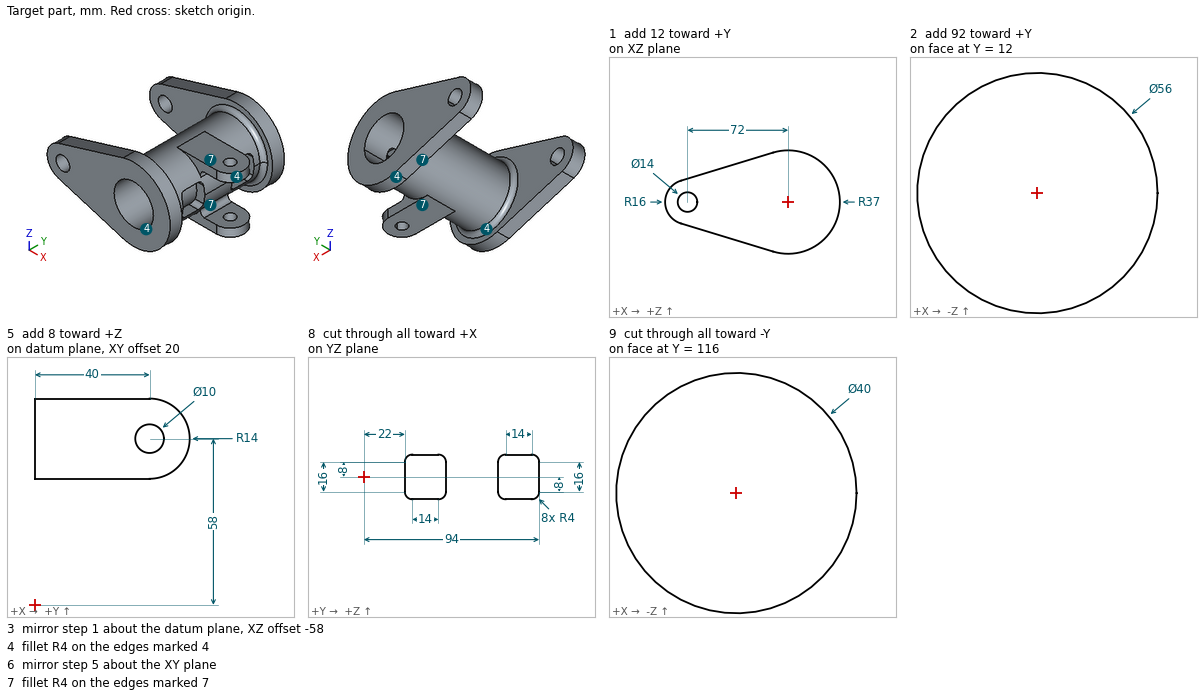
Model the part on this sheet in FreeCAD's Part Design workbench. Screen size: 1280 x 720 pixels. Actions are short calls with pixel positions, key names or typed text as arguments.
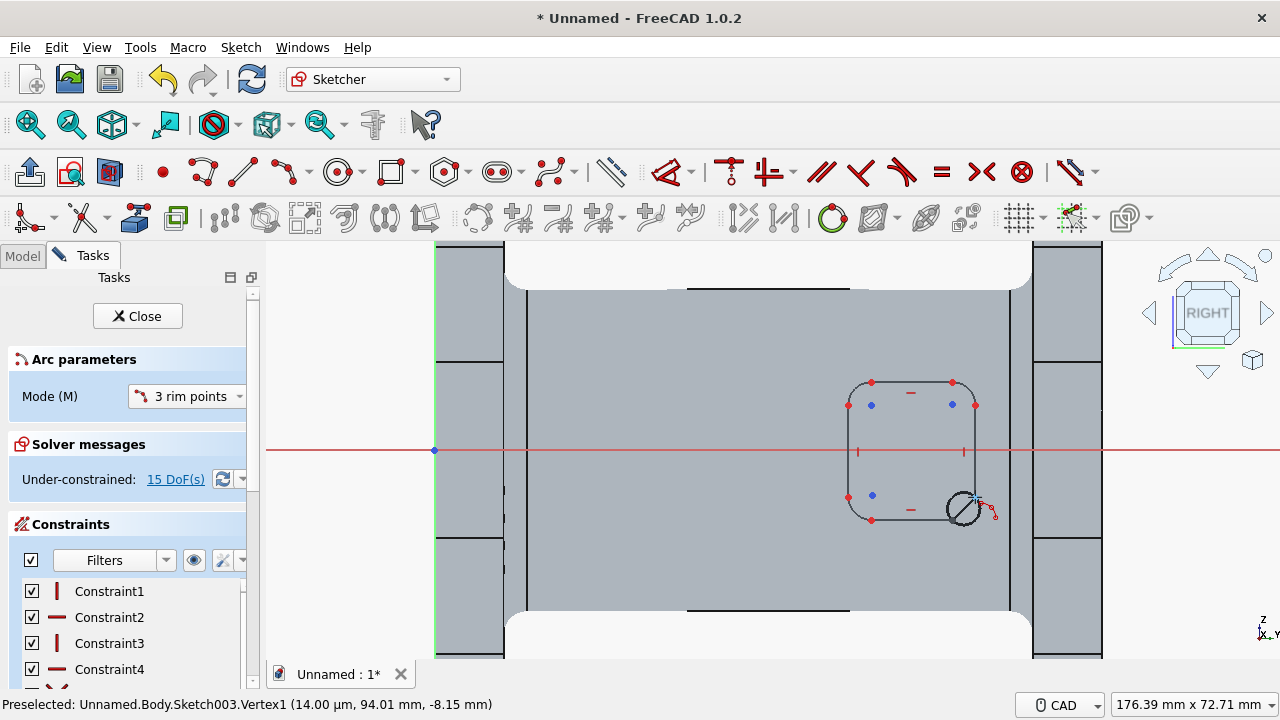
scroll(968, 513, up, 5)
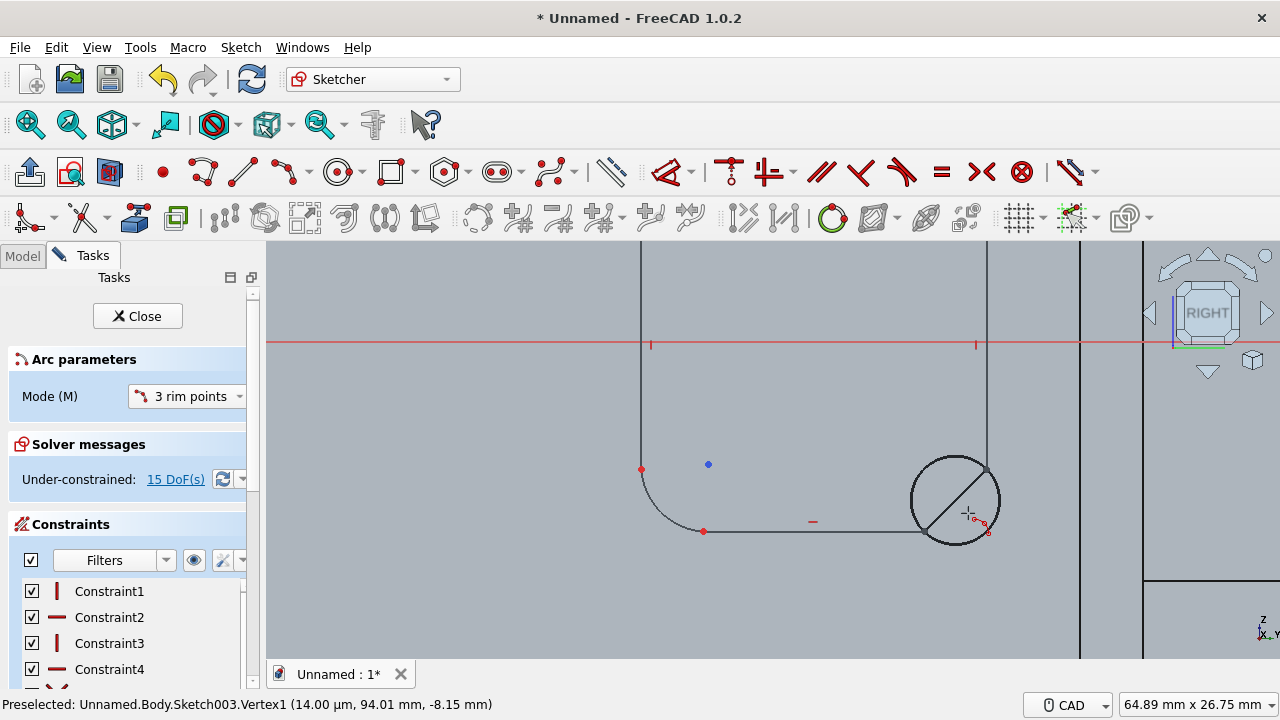
click(968, 511)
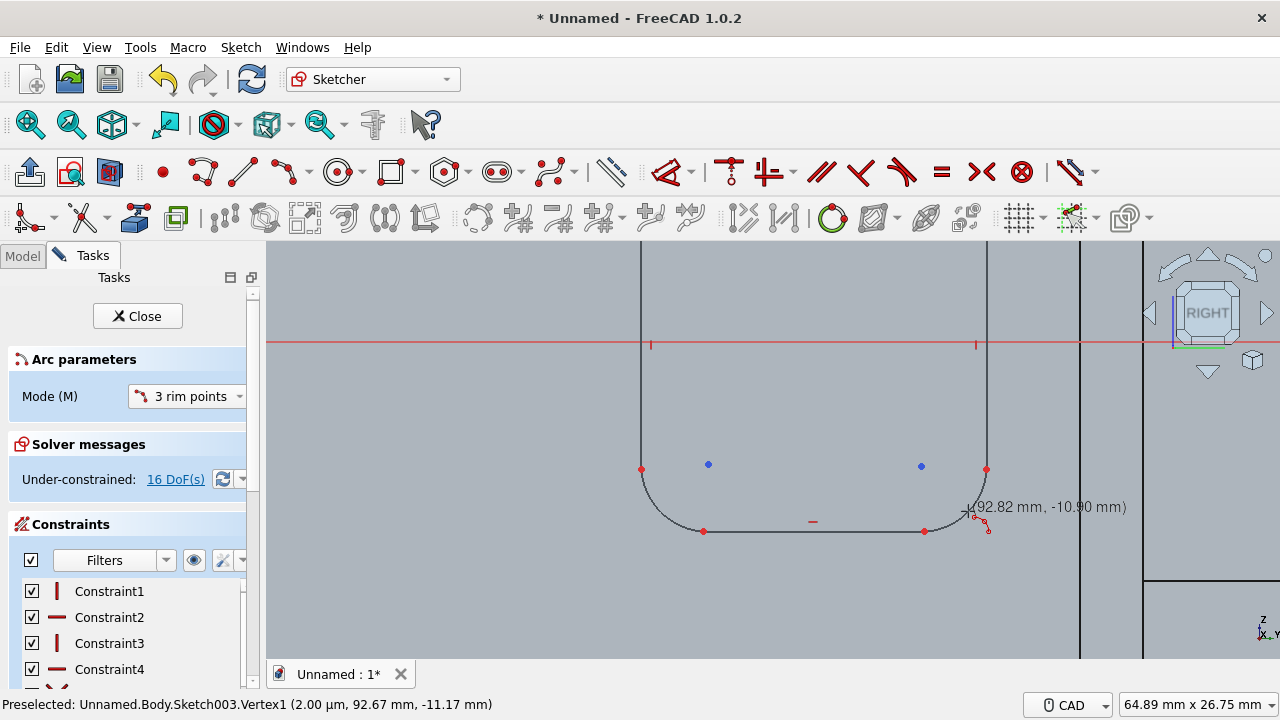
click(244, 172)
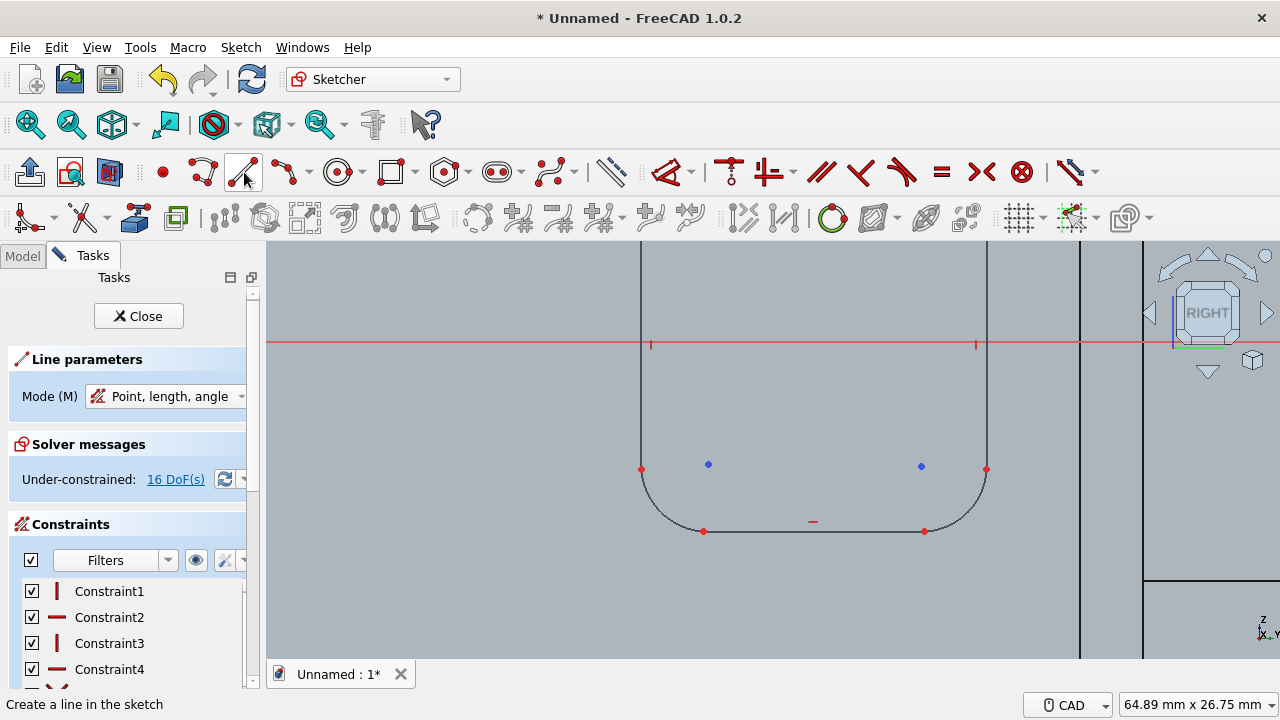
scroll(968, 513, down, 5)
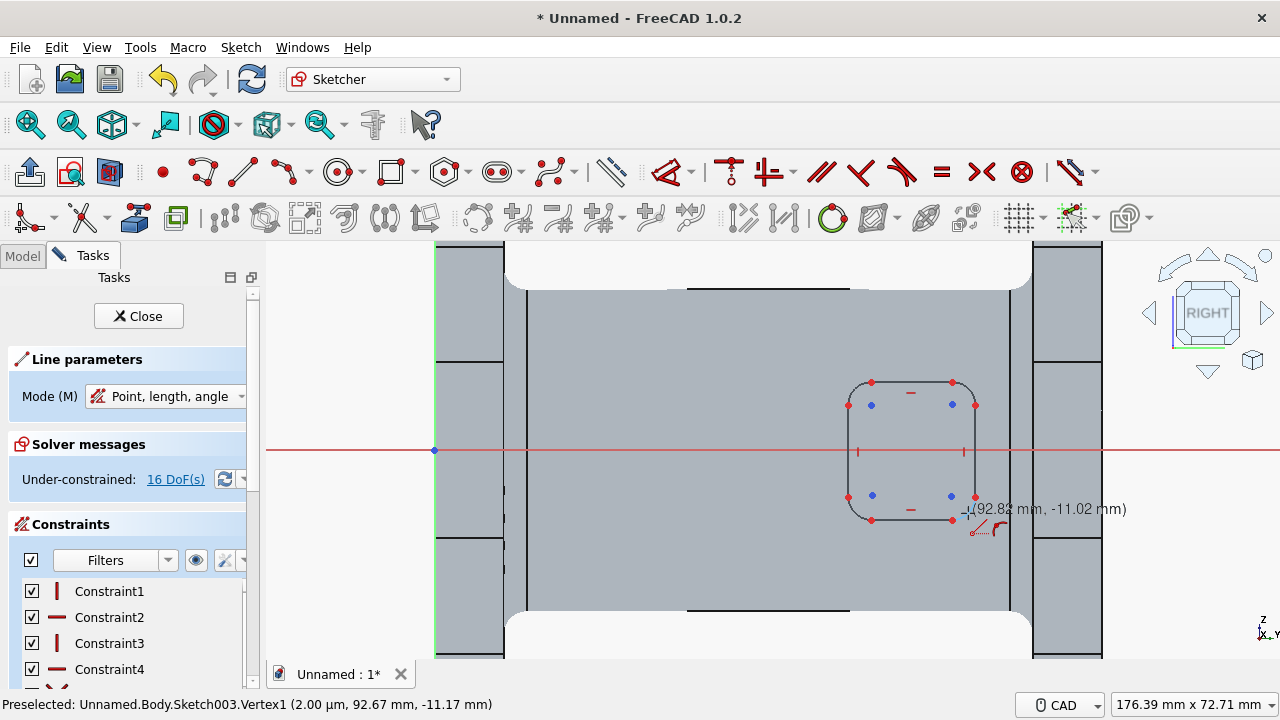
click(561, 404)
click(561, 496)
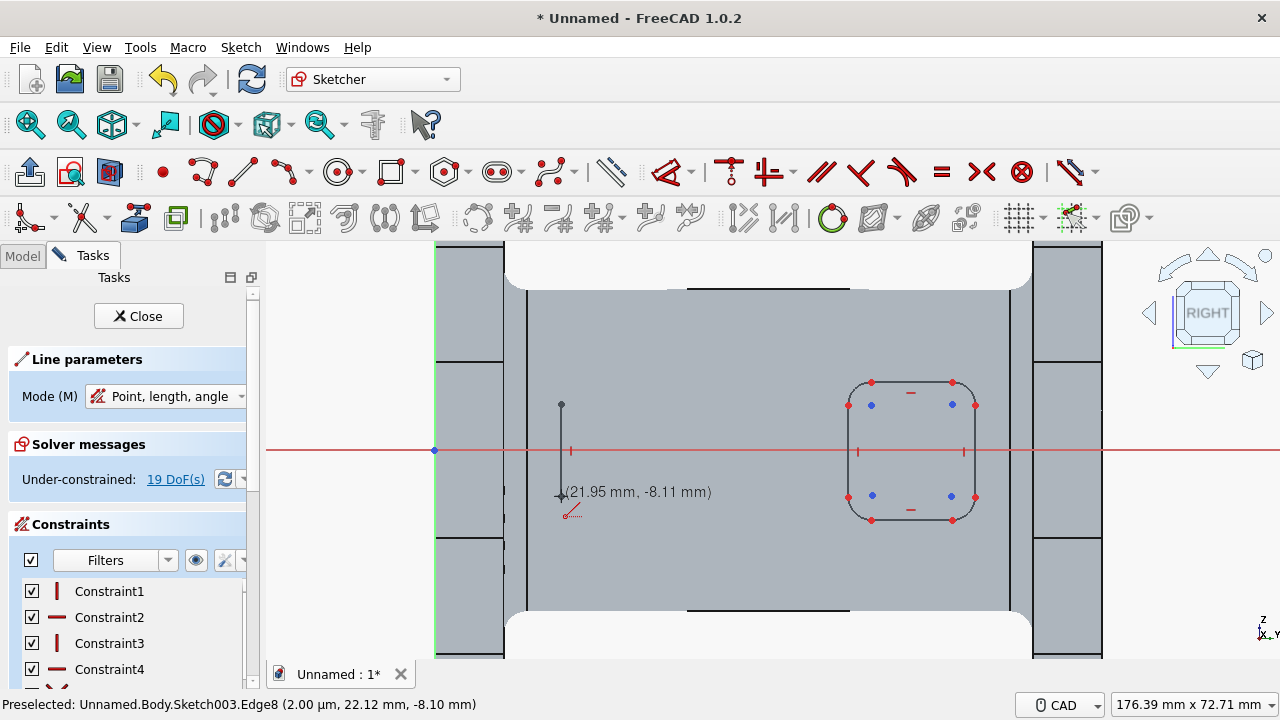
click(584, 519)
click(665, 519)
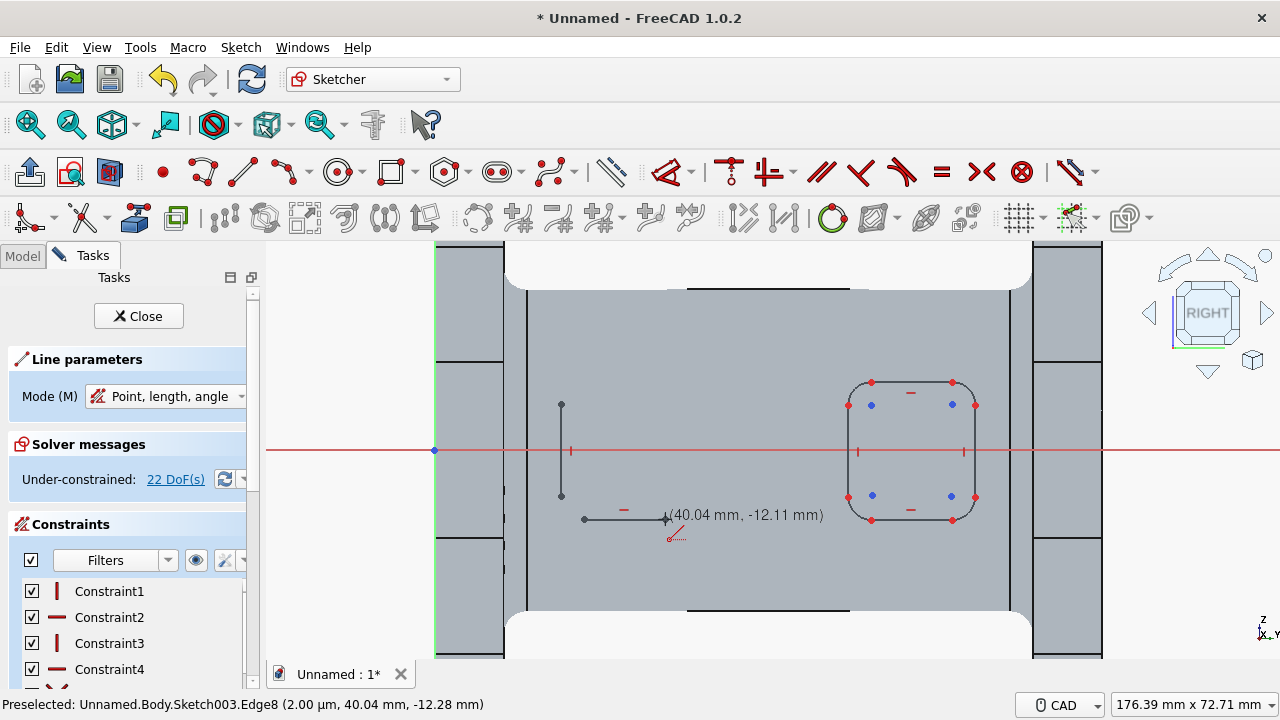
click(688, 496)
click(688, 404)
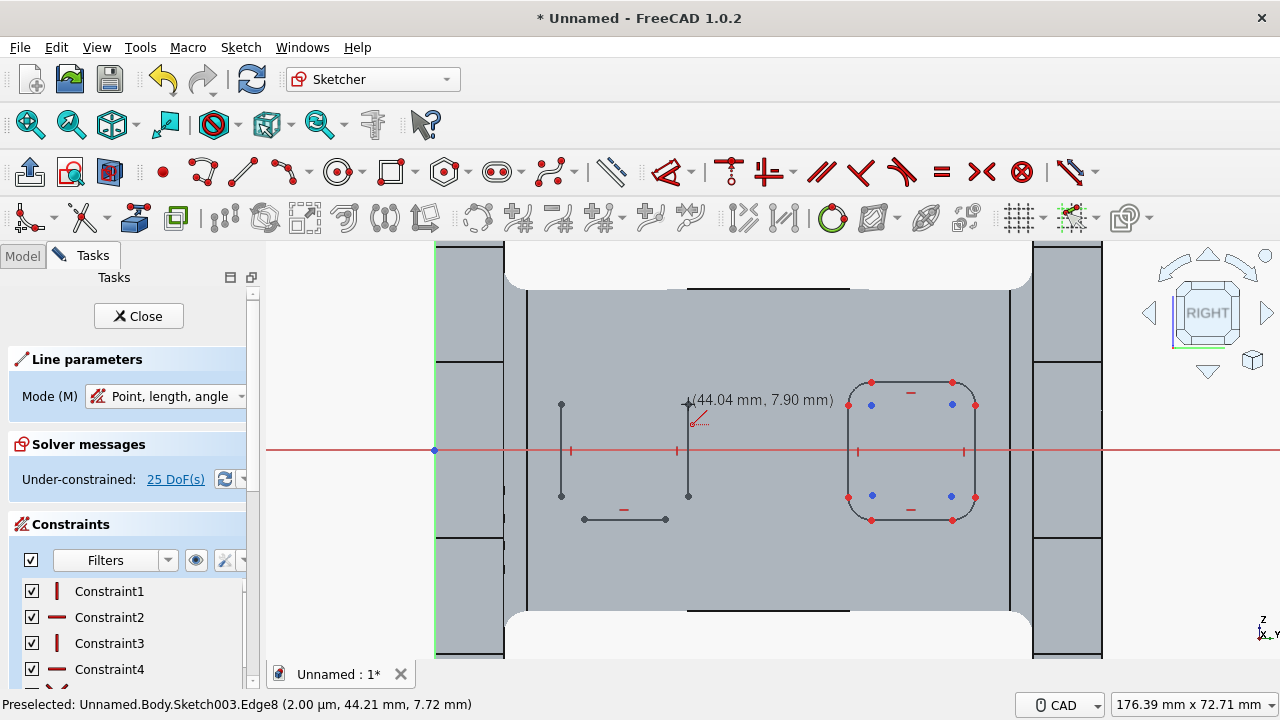
click(665, 381)
click(584, 381)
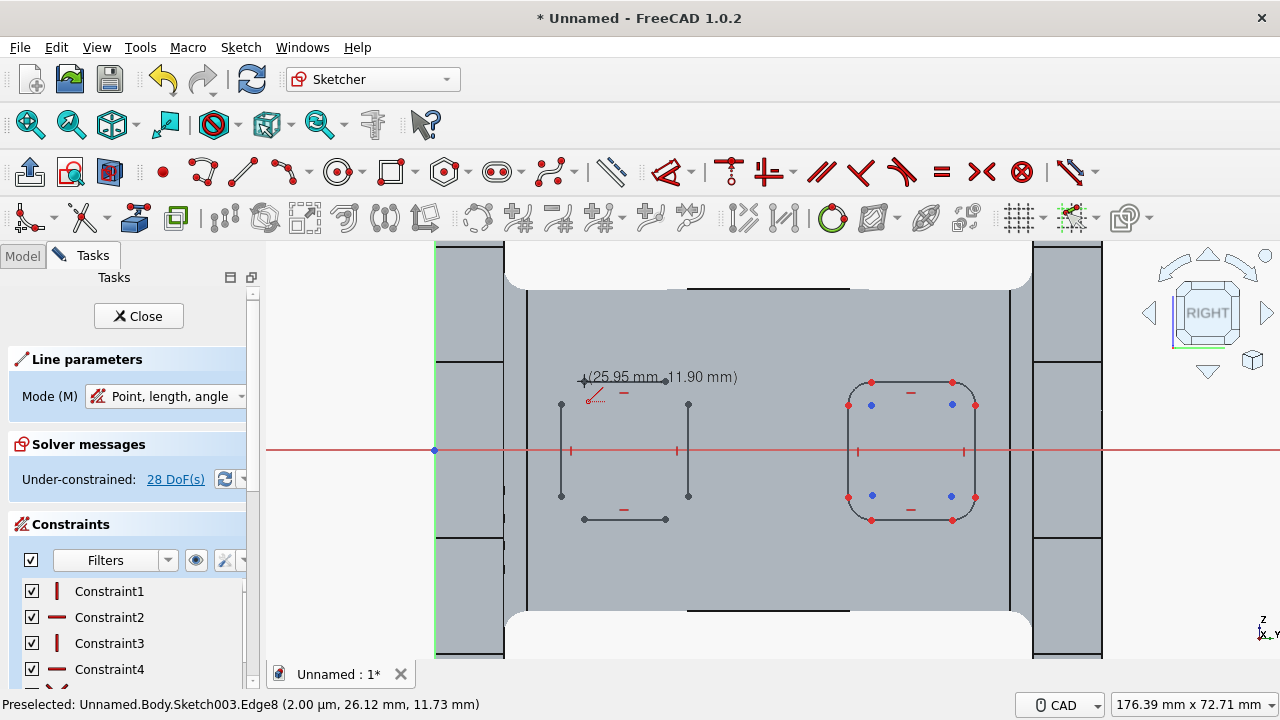
click(284, 172)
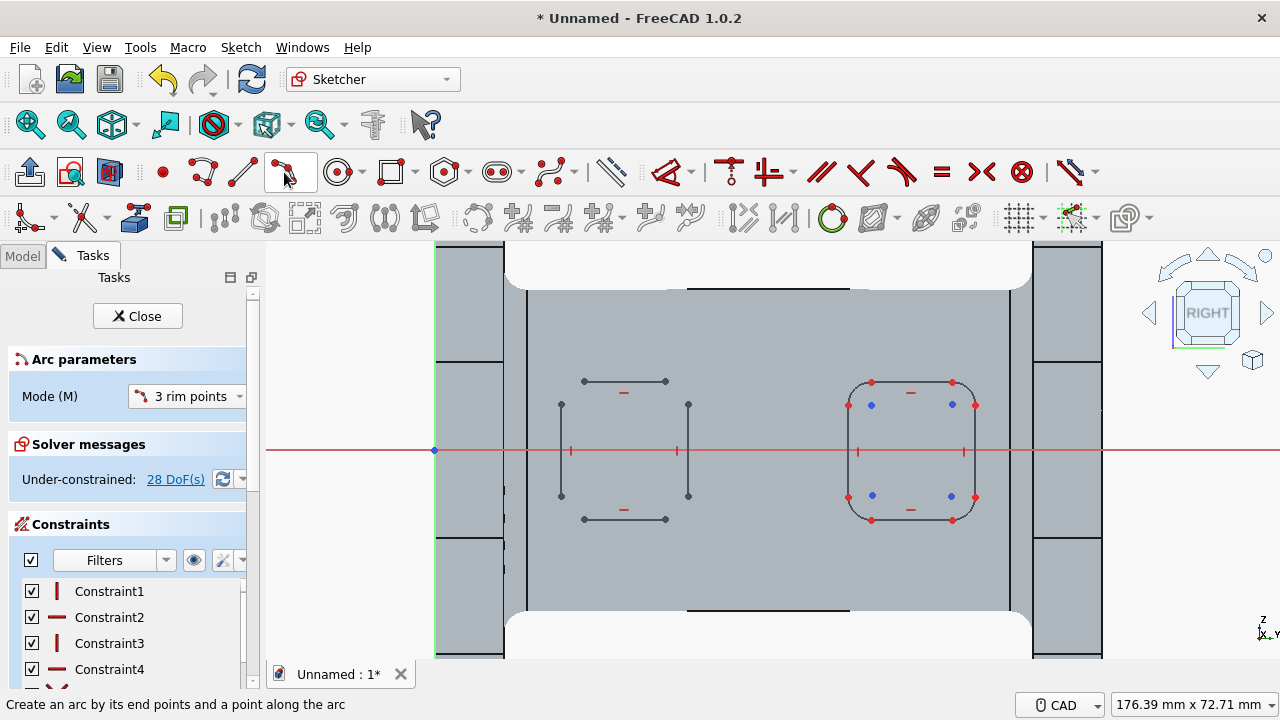
click(561, 497)
click(584, 520)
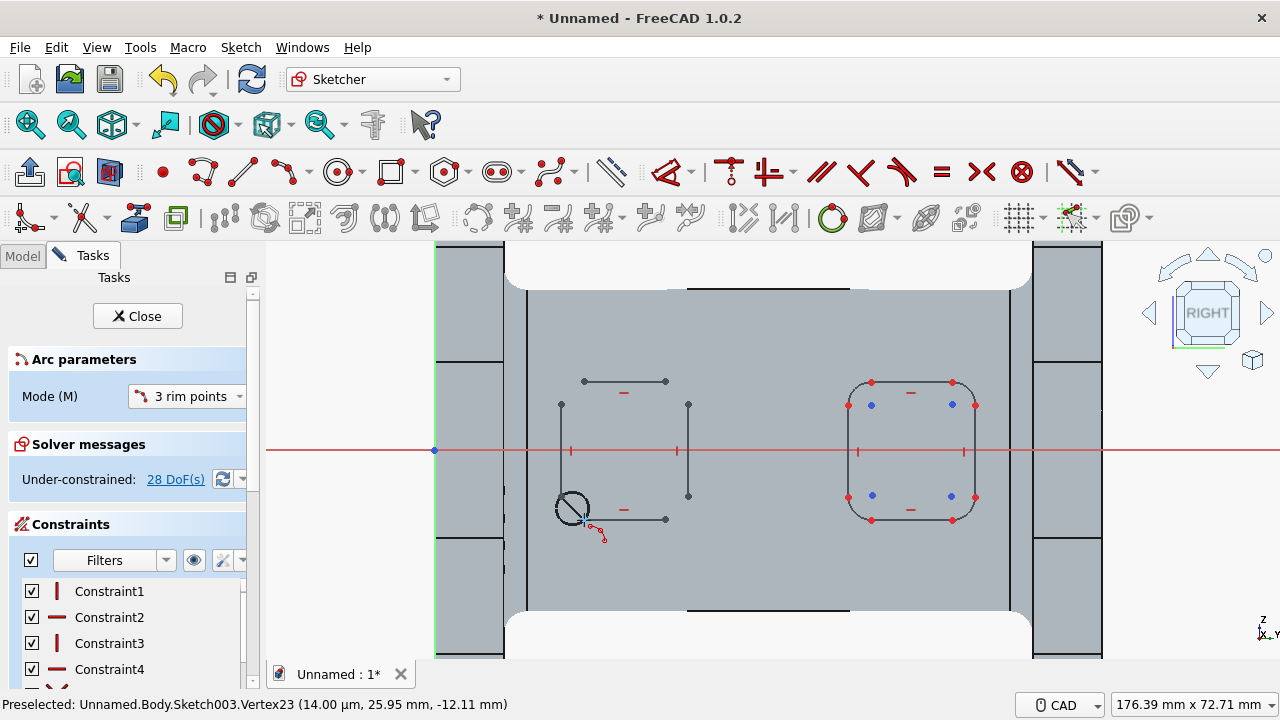
scroll(568, 513, up, 5)